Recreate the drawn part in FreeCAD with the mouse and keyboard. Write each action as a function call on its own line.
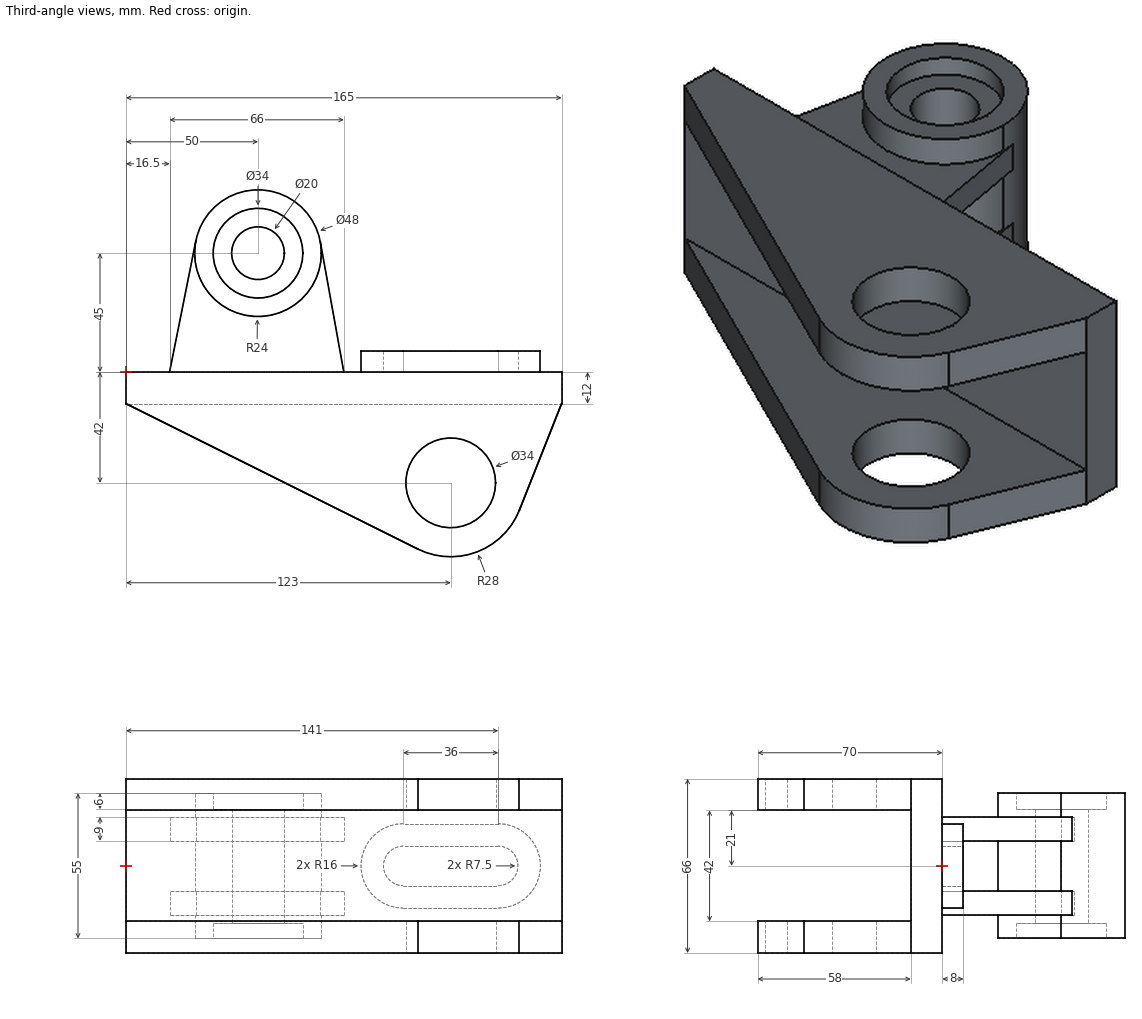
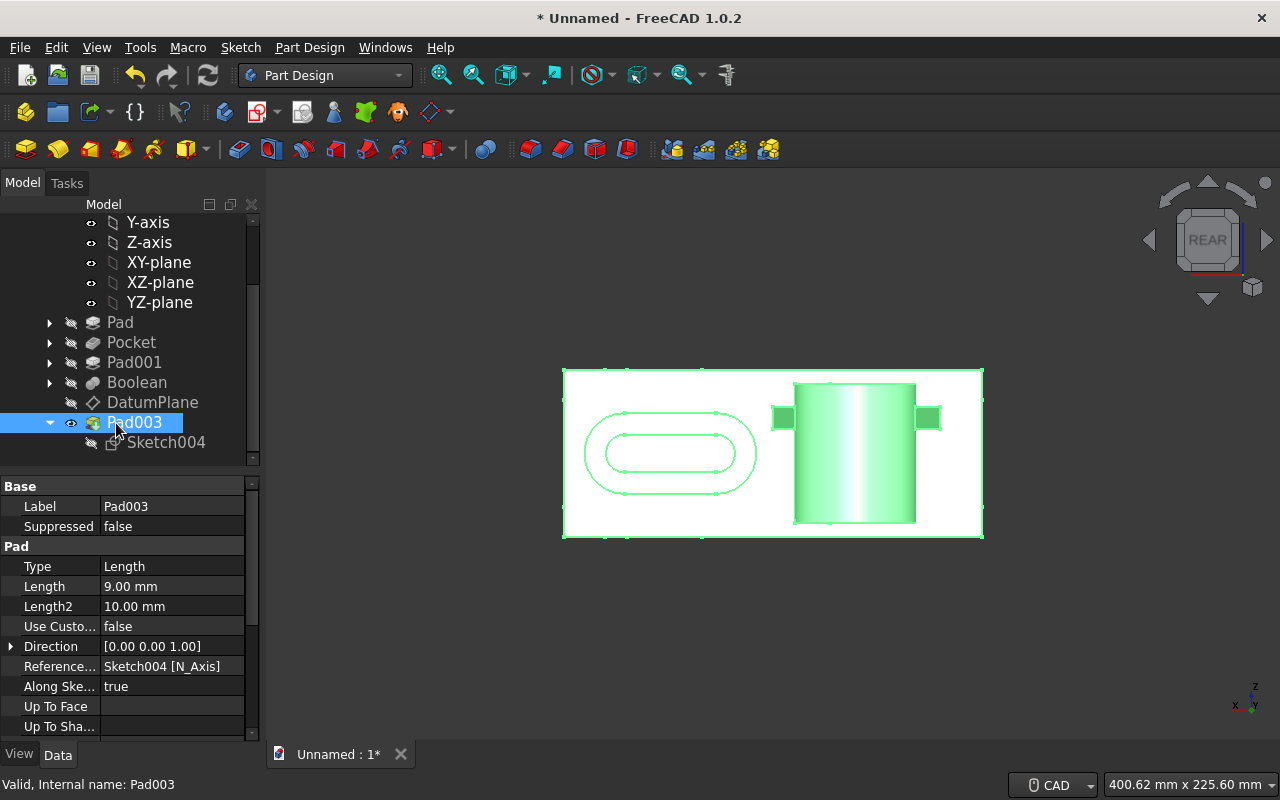
click(672, 150)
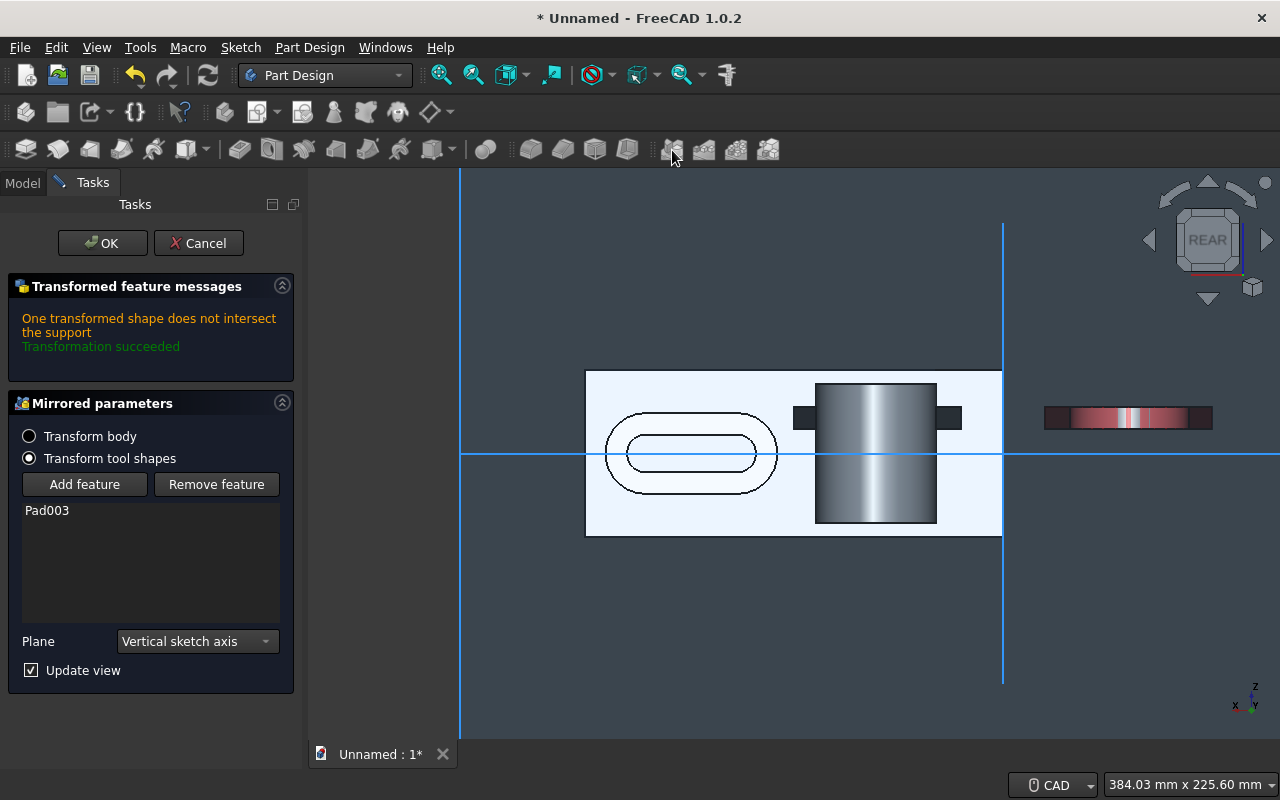
click(198, 642)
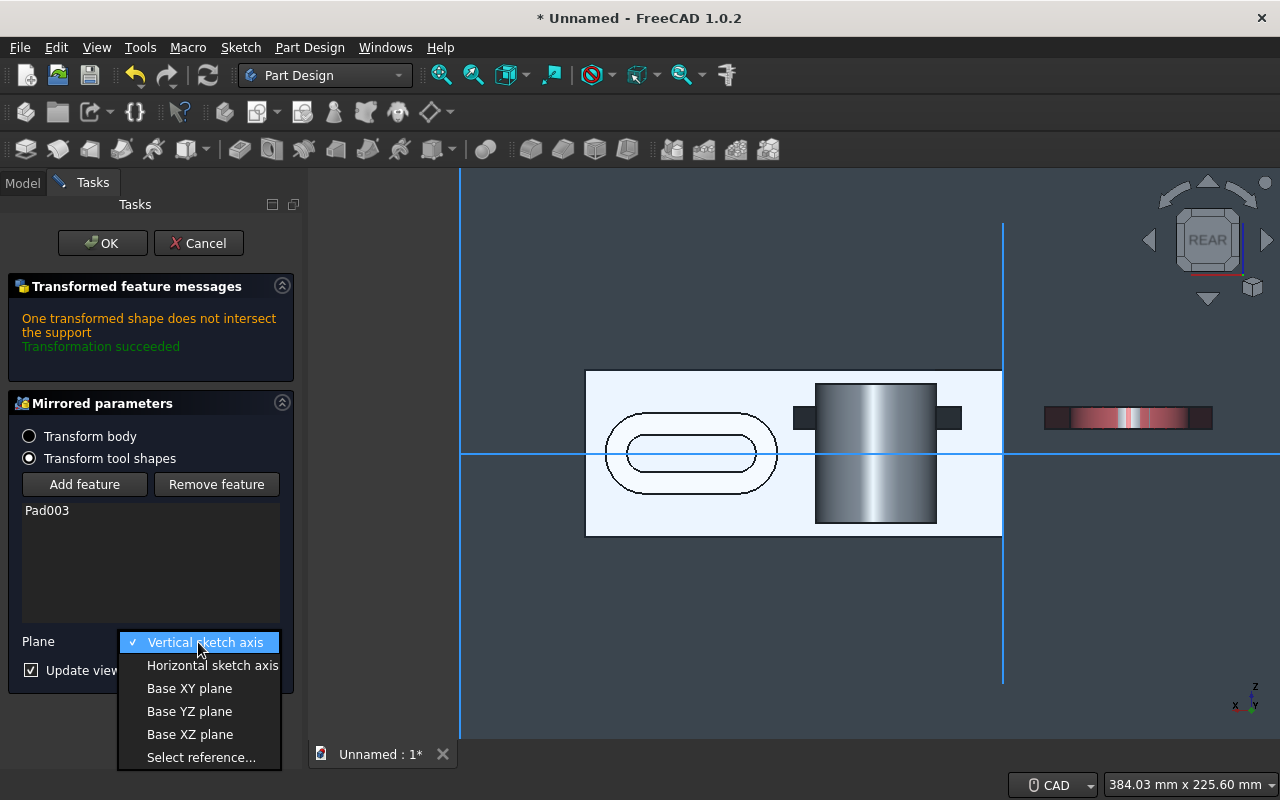
click(198, 688)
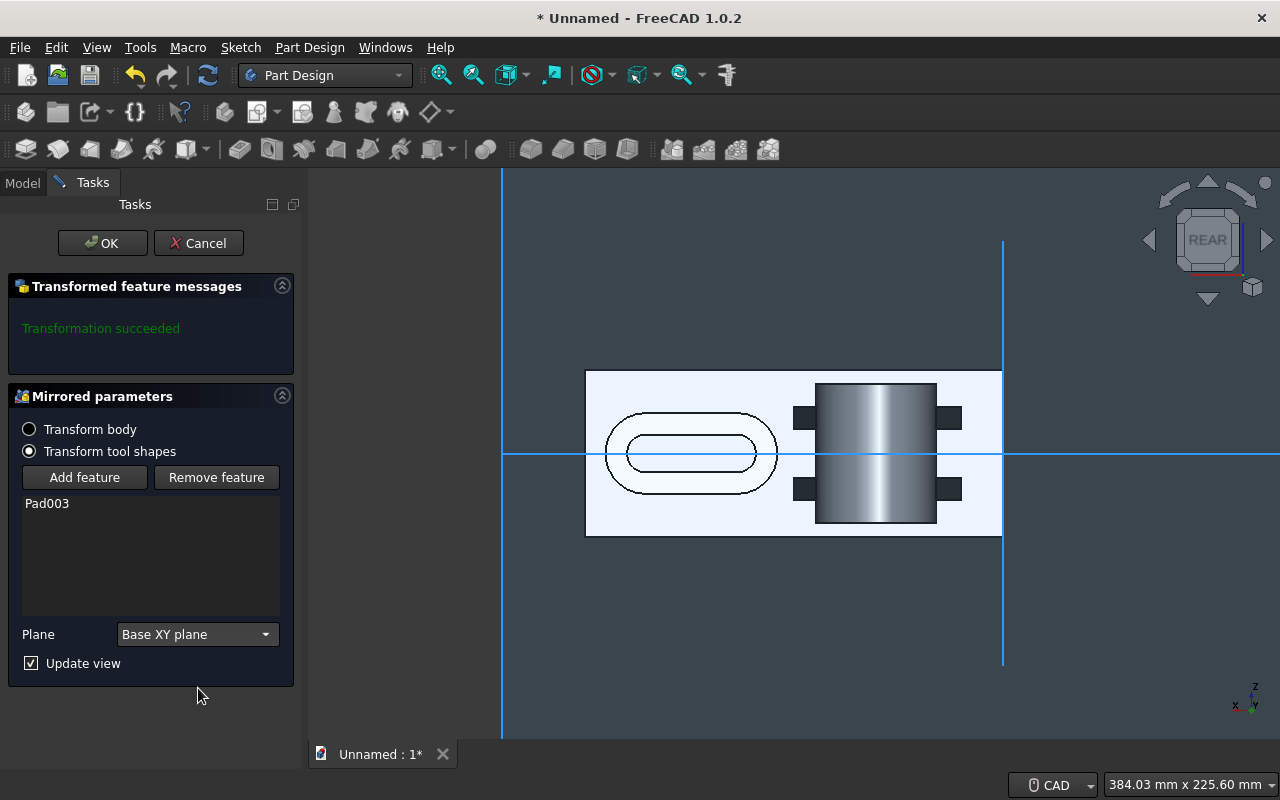
click(103, 243)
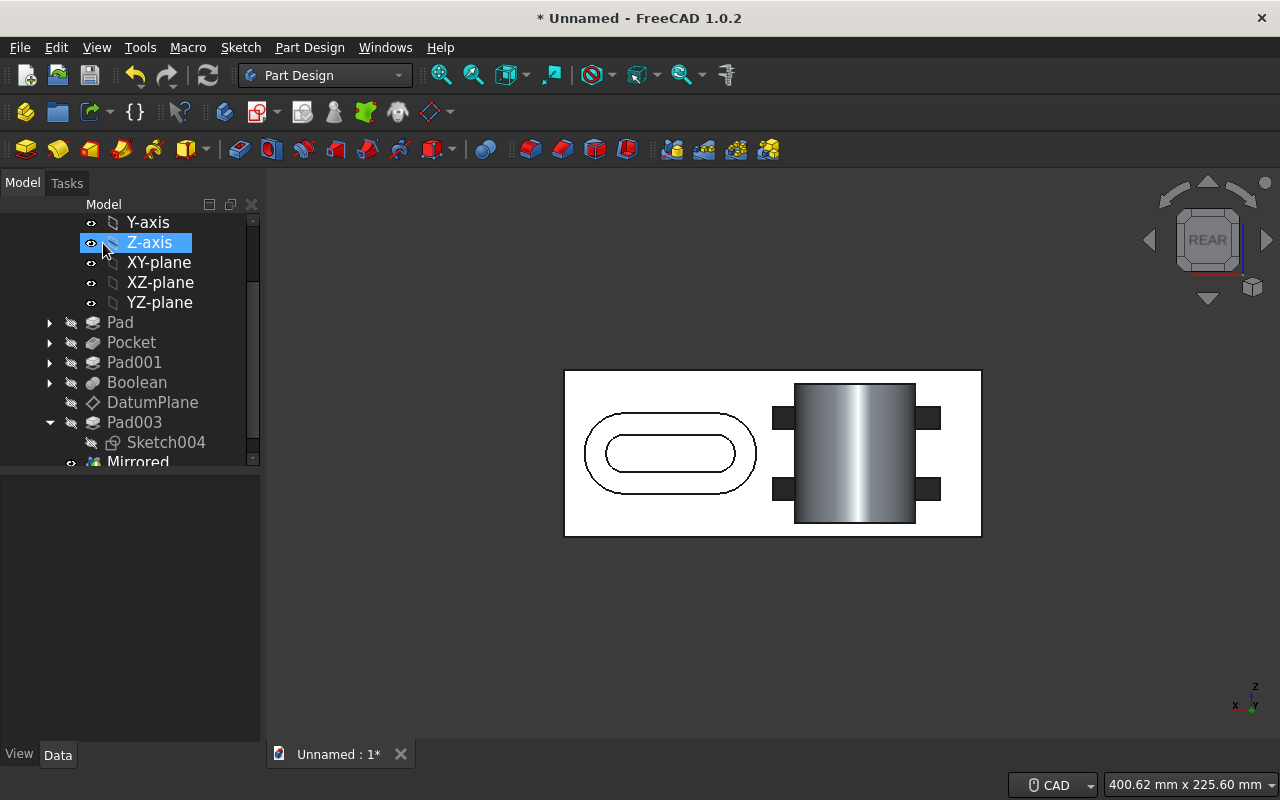
key(v)
key(f)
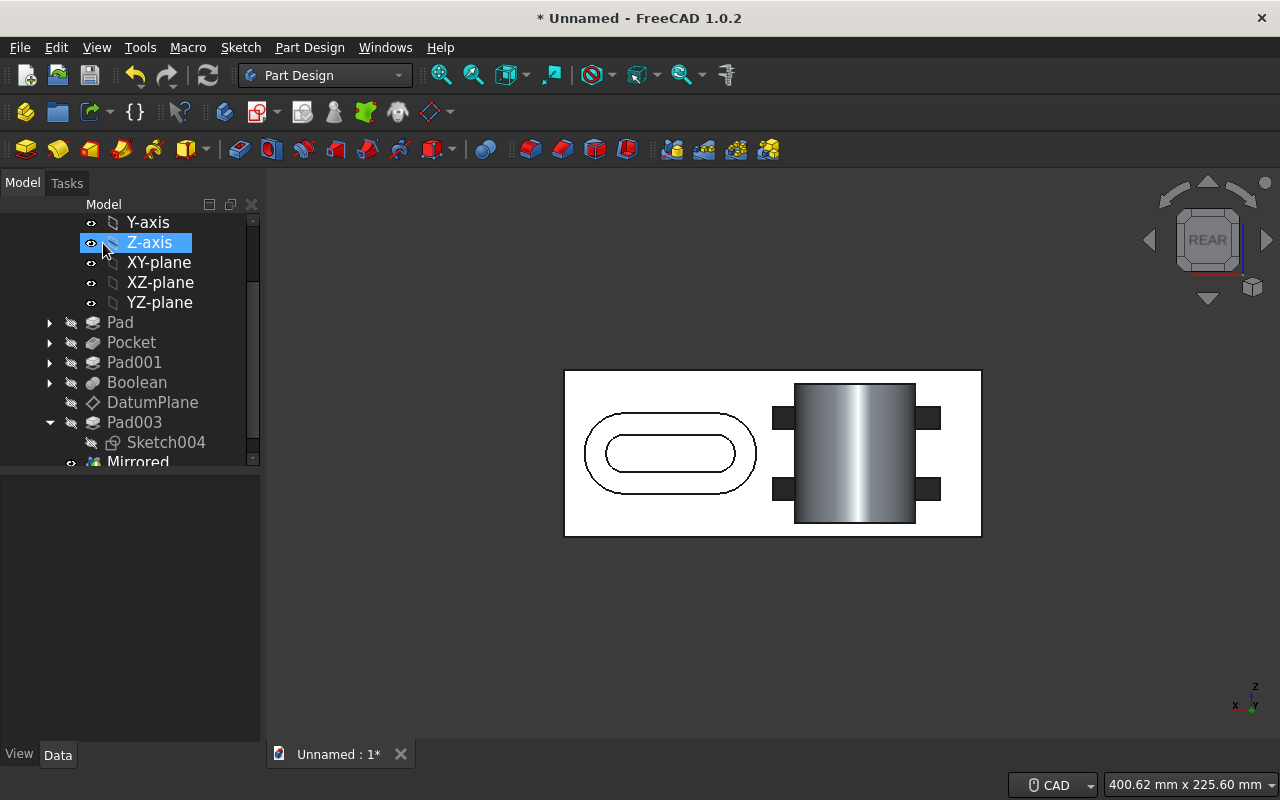
key(0)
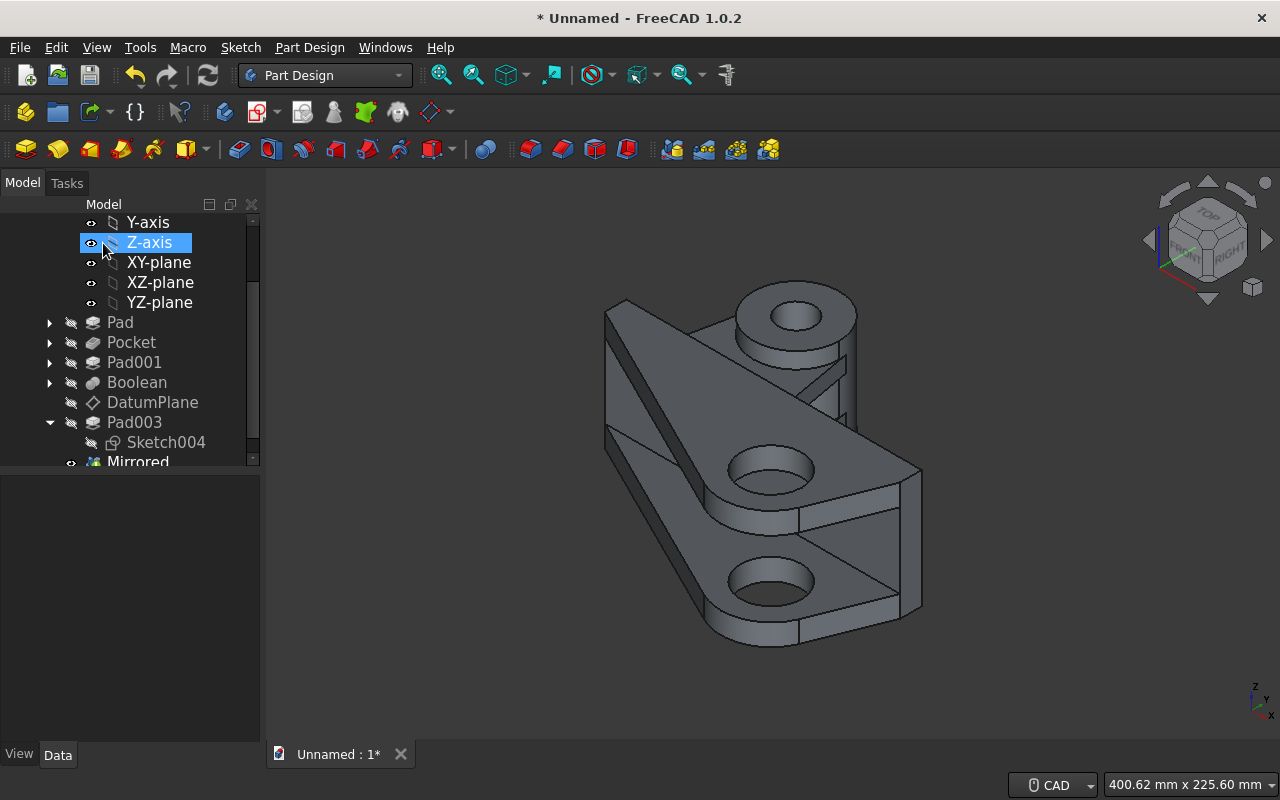
click(759, 322)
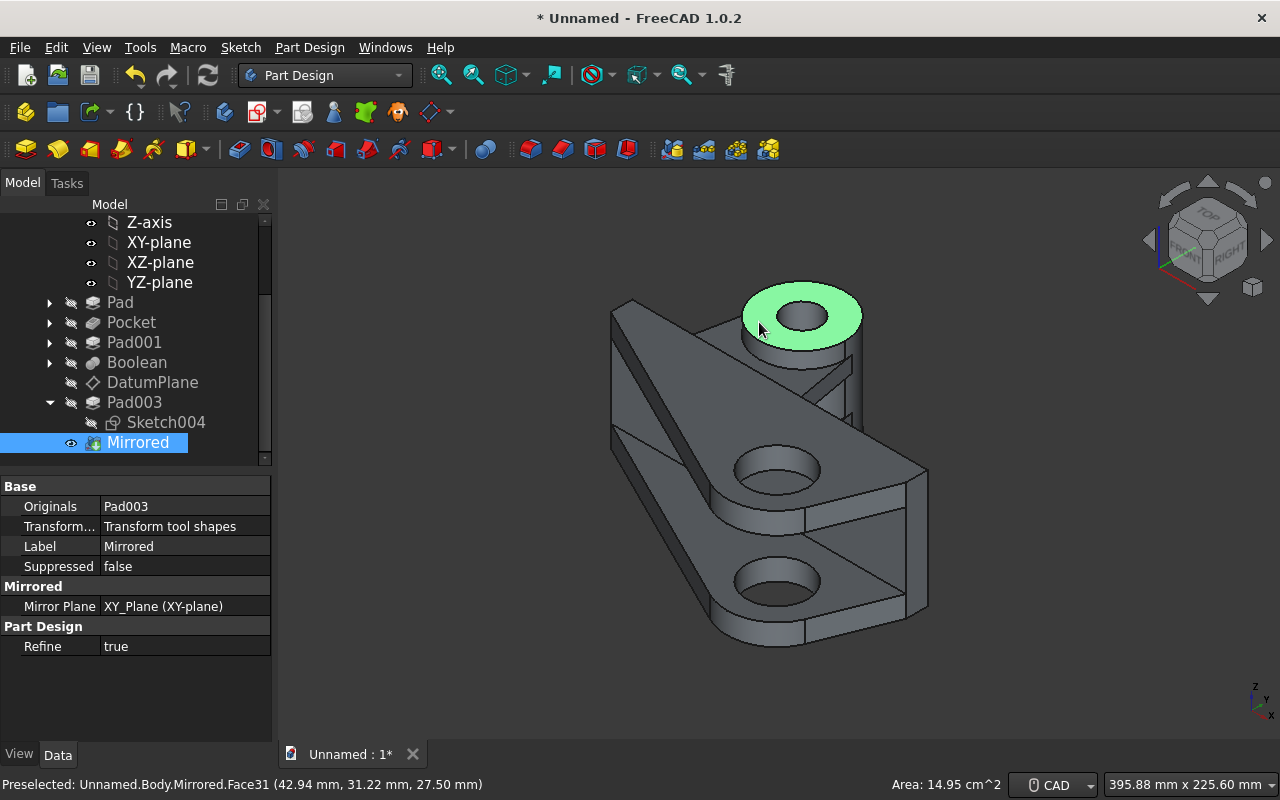
click(258, 112)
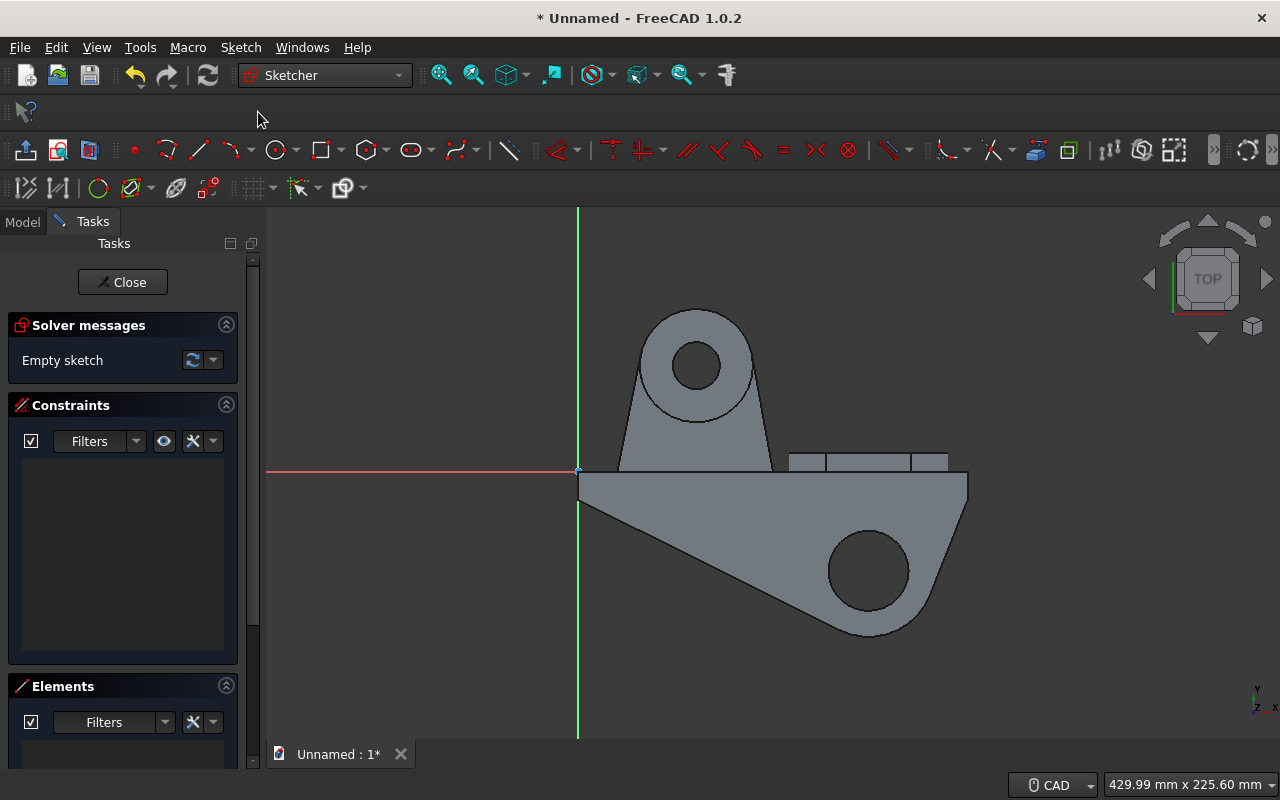
scroll(619, 338, up, 4)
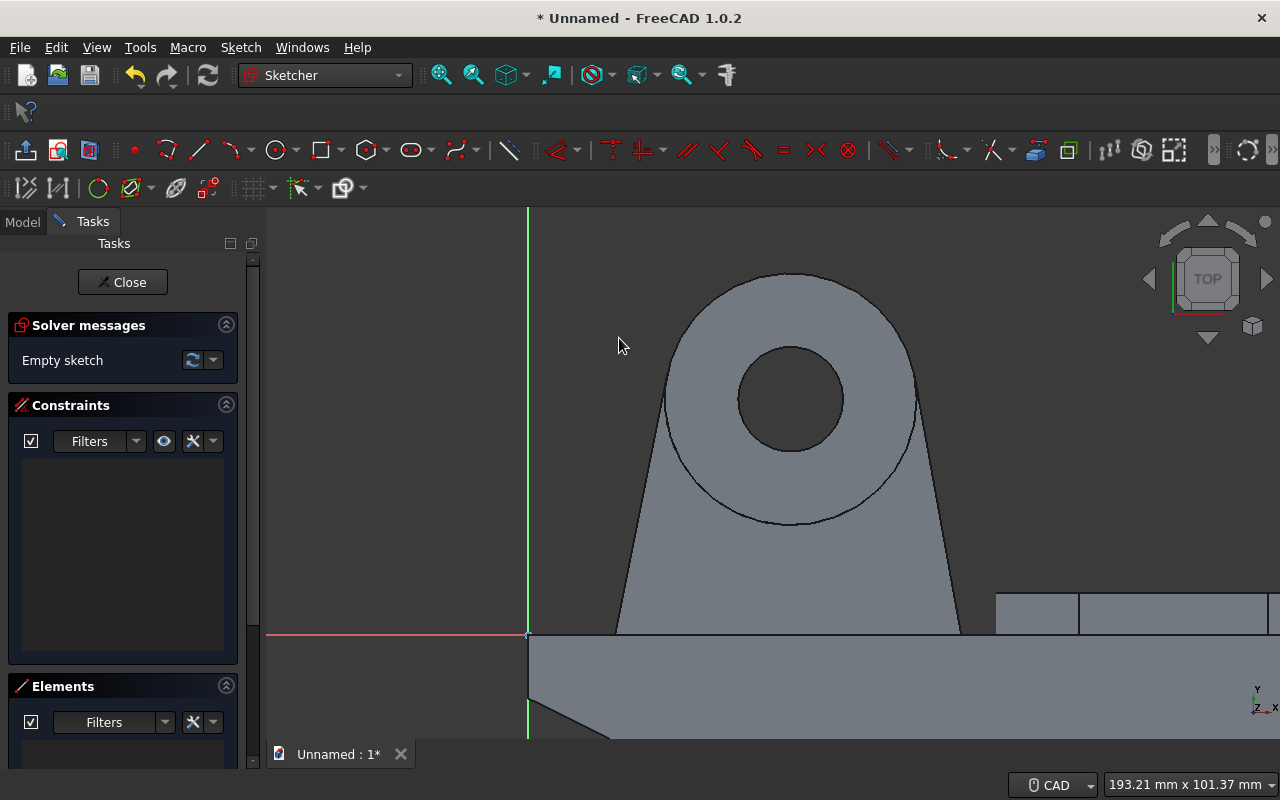
key(g)
key(c)